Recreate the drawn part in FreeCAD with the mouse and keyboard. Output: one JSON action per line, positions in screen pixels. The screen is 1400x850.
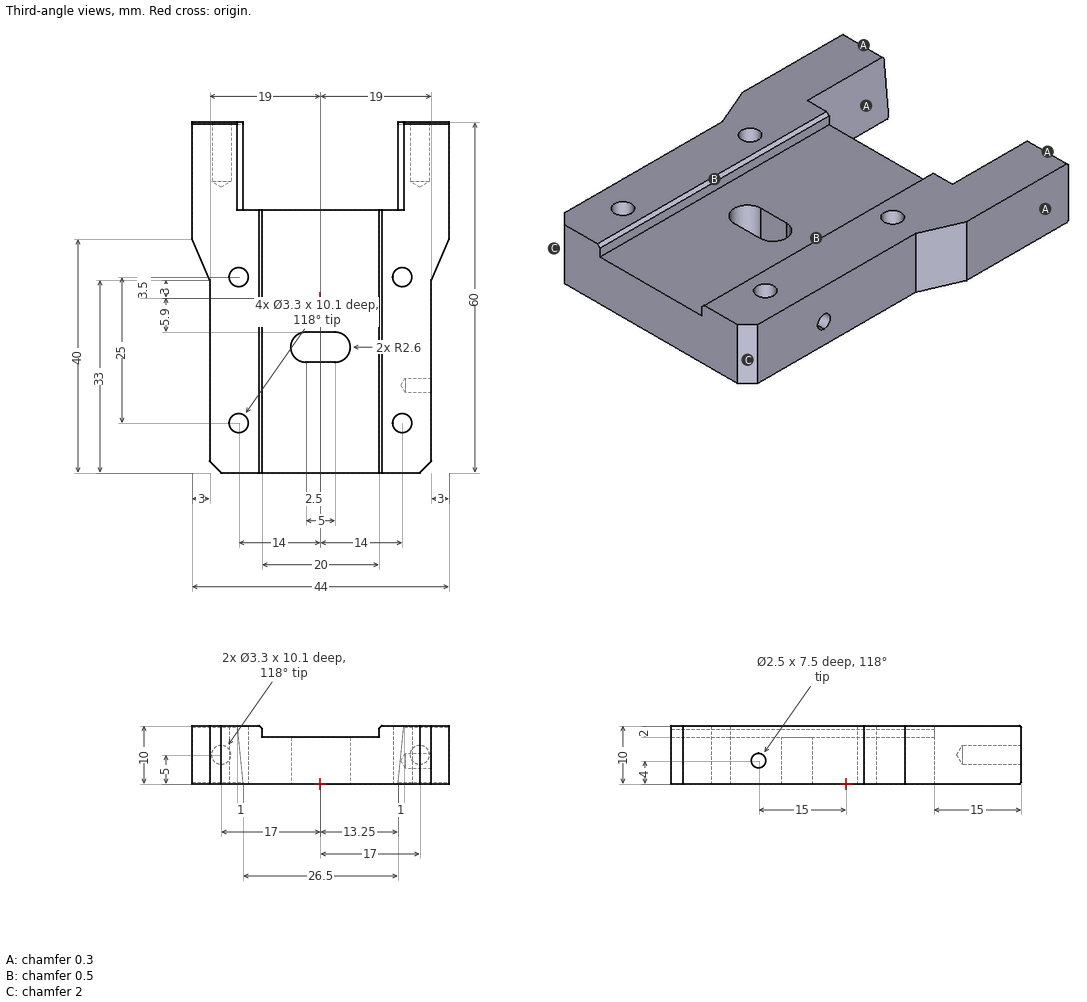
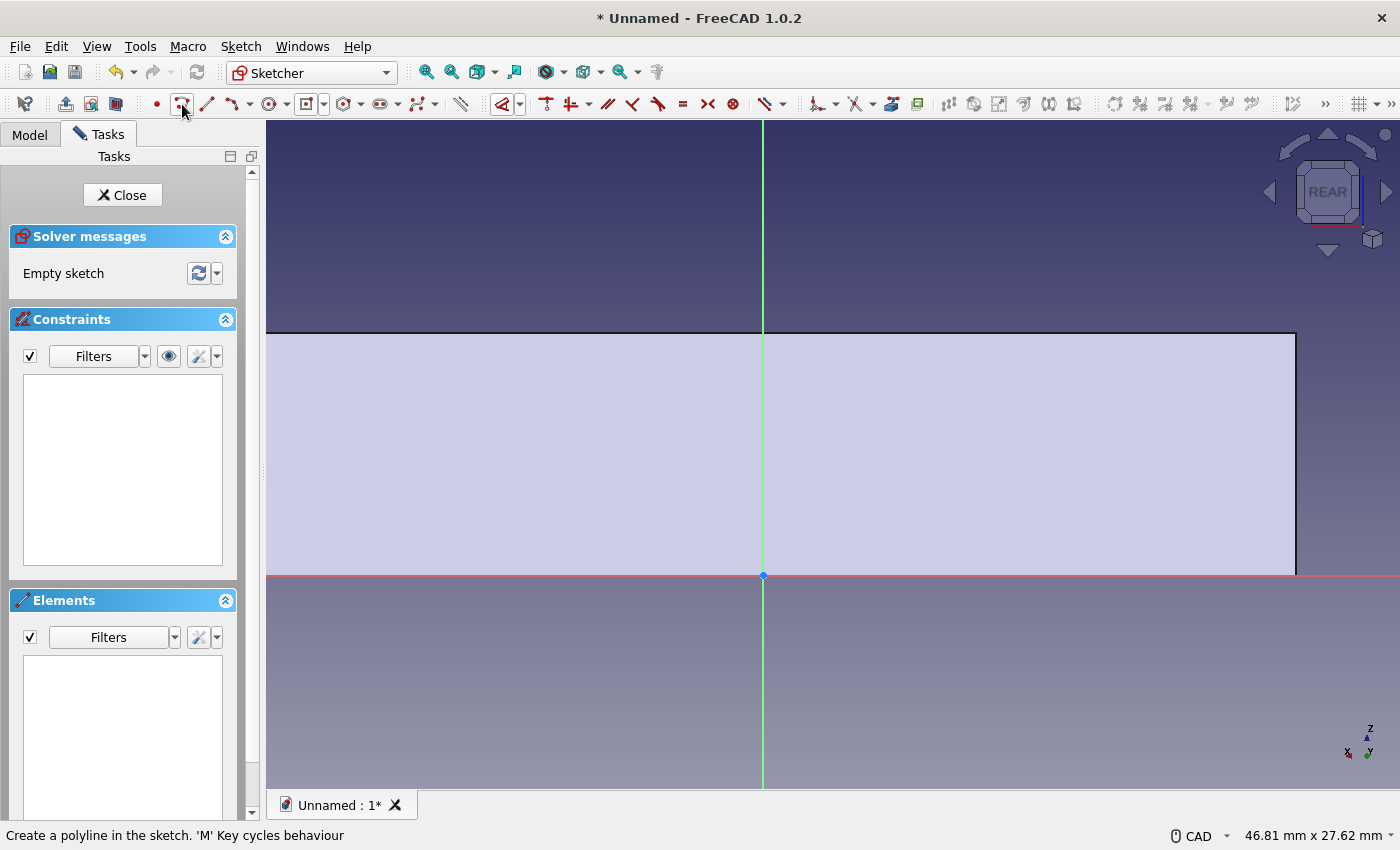
{"action": "left_click", "coordinate": [442, 576]}
{"action": "left_click", "coordinate": [1084, 567]}
{"action": "left_click", "coordinate": [1109, 333]}
{"action": "left_click", "coordinate": [418, 333]}
{"action": "left_click", "coordinate": [442, 576]}
{"action": "key", "text": "Escape"}
{"action": "key", "text": "Escape"}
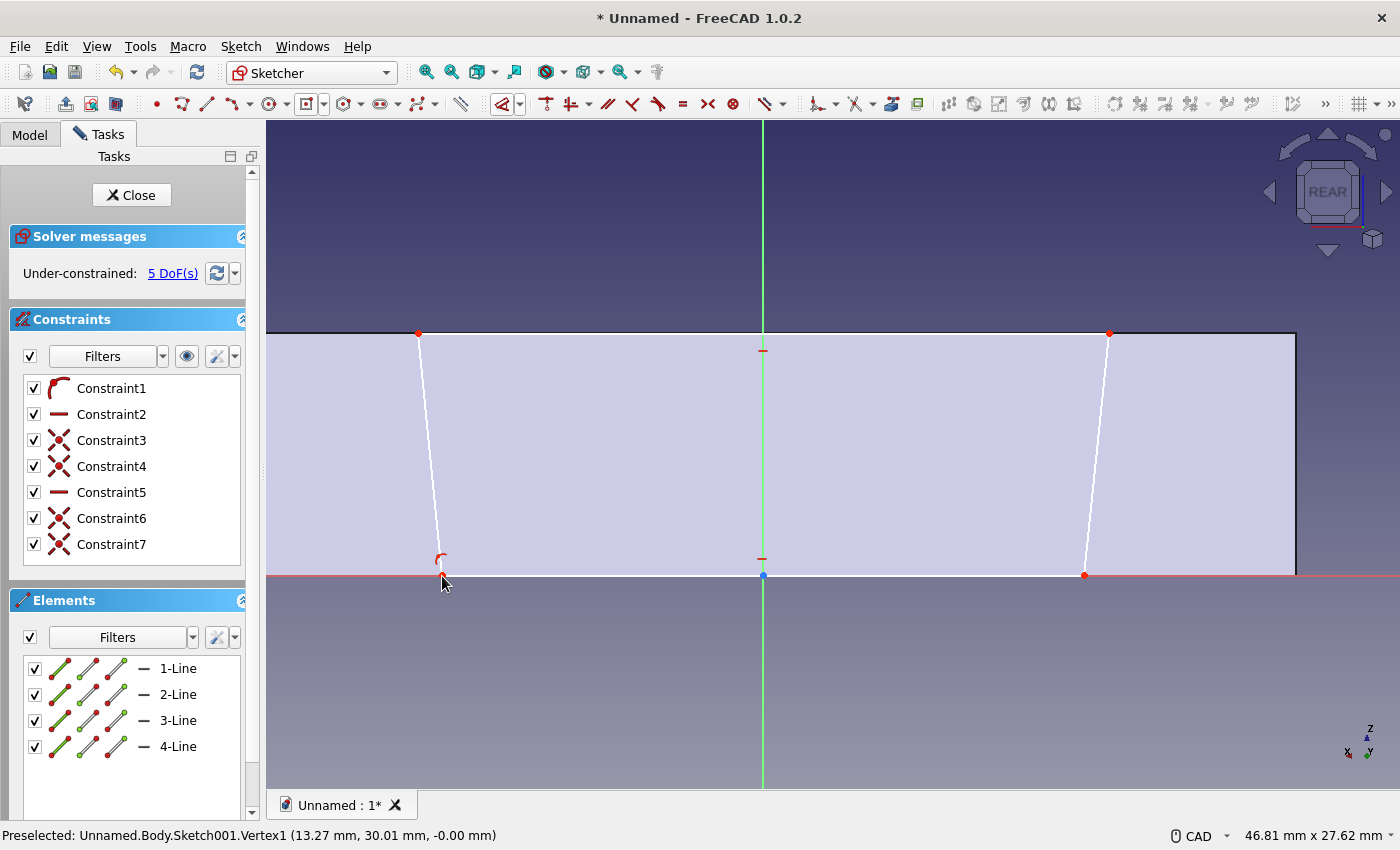
{"action": "scroll", "coordinate": [1091, 503], "scroll_direction": "up", "scroll_amount": 3}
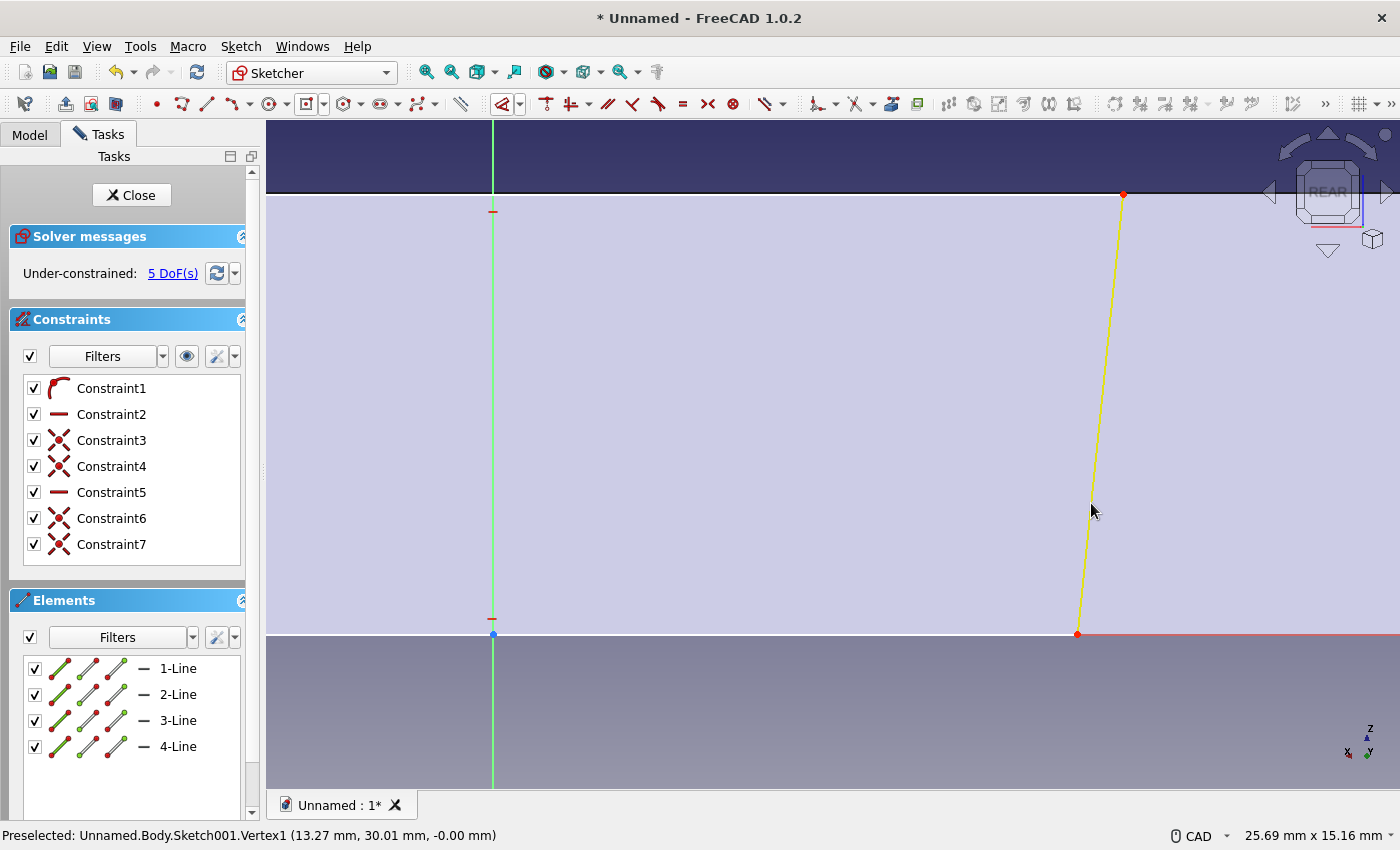
{"action": "left_click", "coordinate": [1091, 503]}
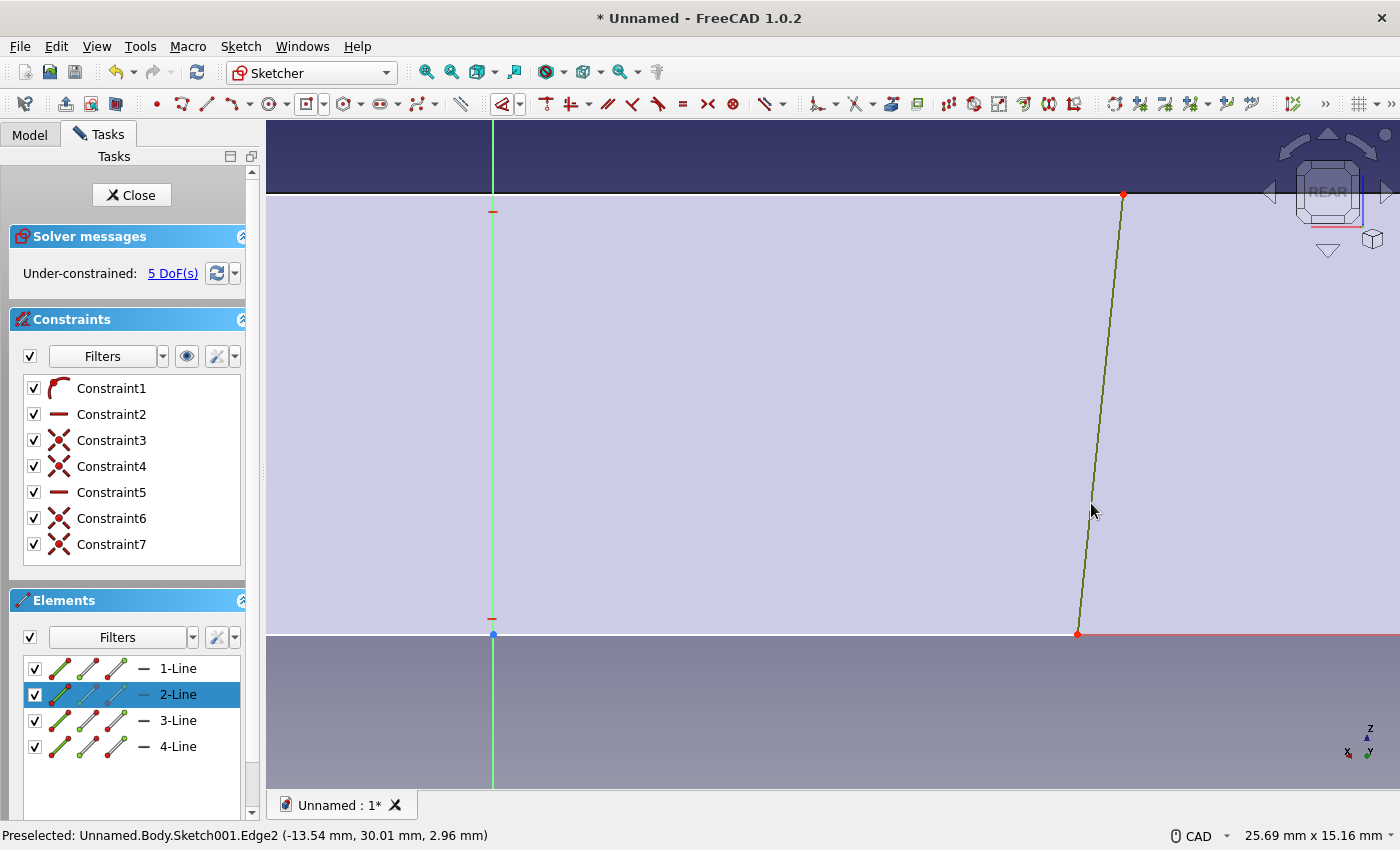
{"action": "key", "text": "l"}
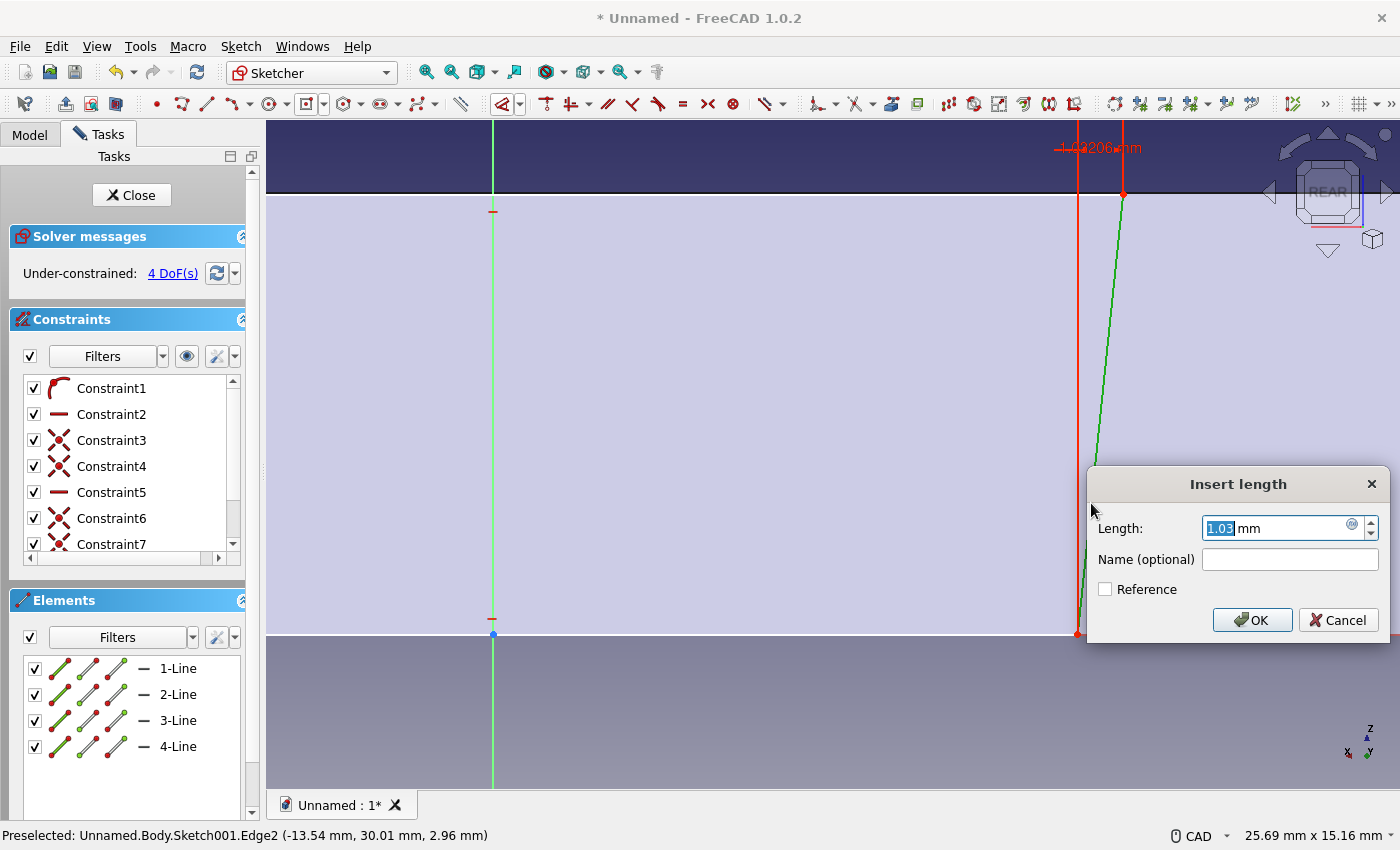
{"action": "type", "text": "1"}
{"action": "key", "text": "Return"}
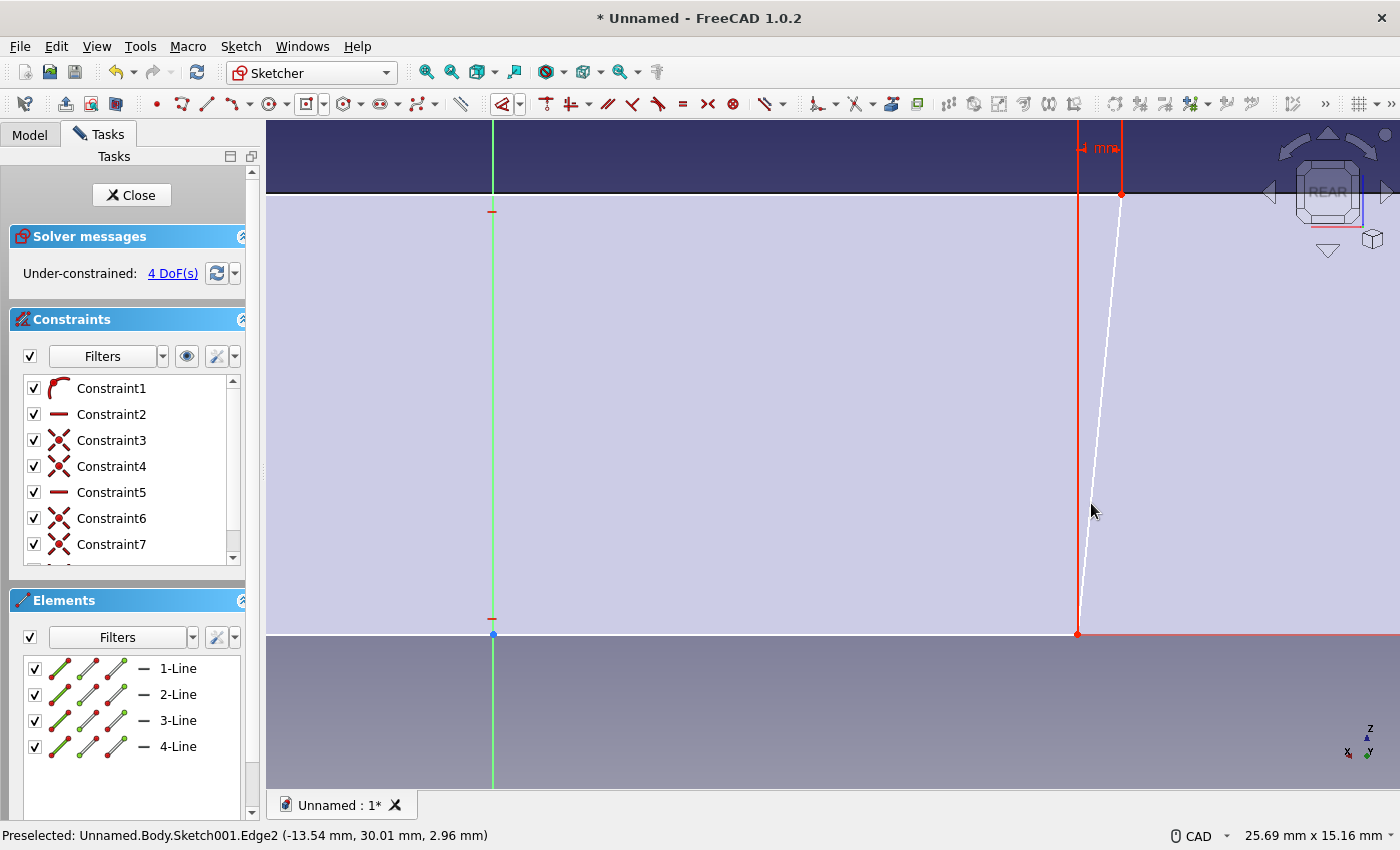
{"action": "scroll", "coordinate": [1094, 504], "scroll_direction": "down", "scroll_amount": 3}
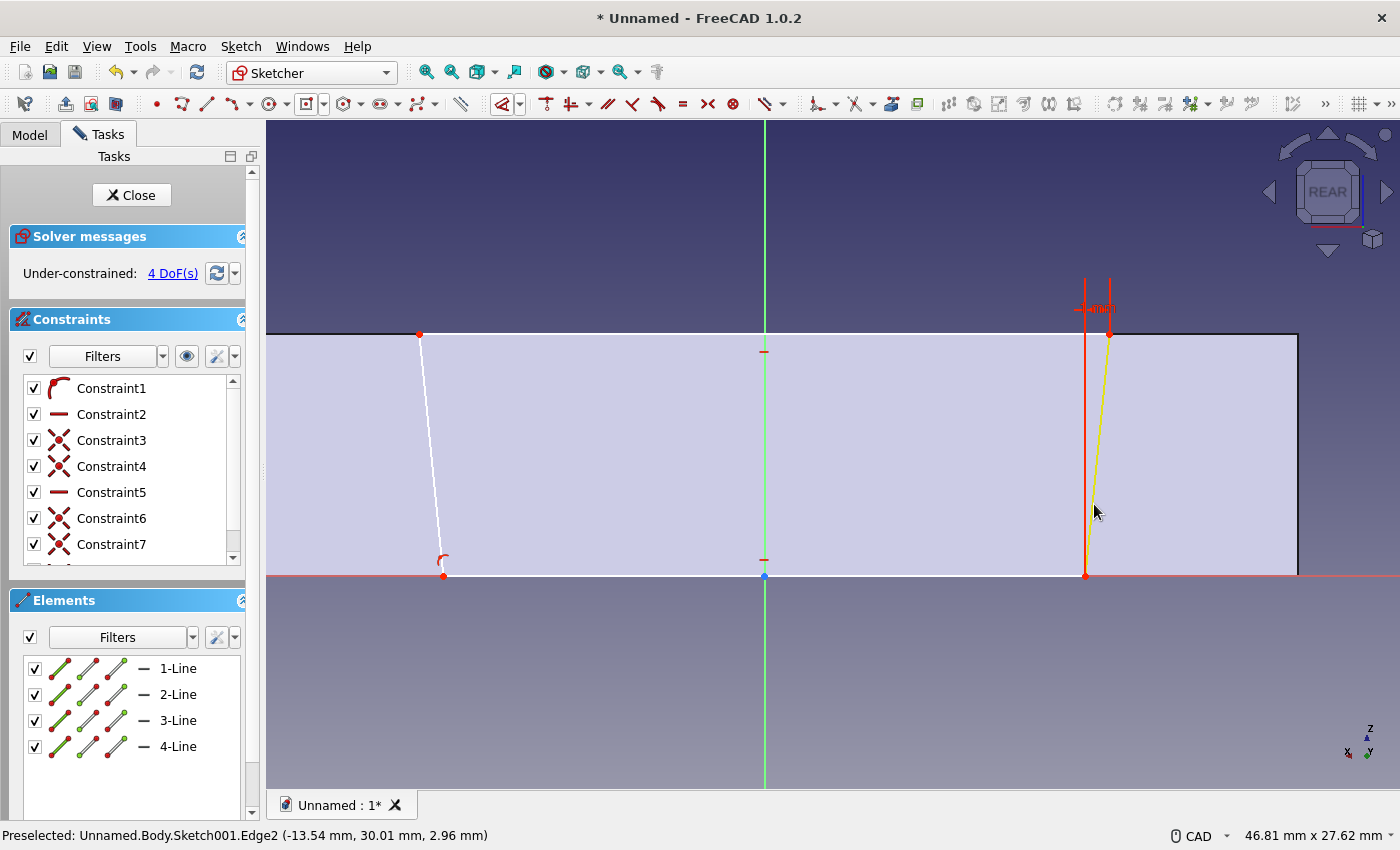
{"action": "scroll", "coordinate": [427, 407], "scroll_direction": "up", "scroll_amount": 3}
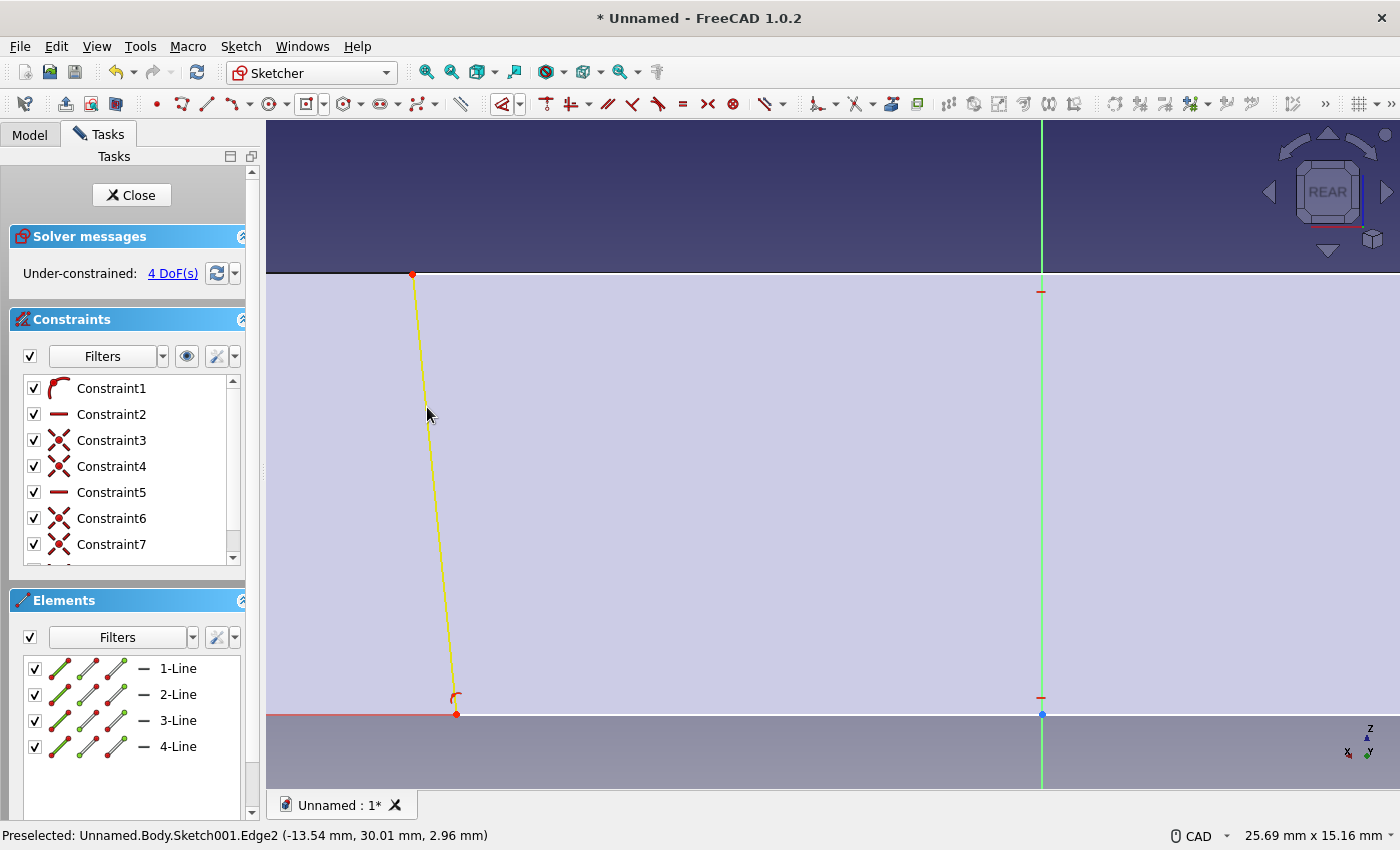
{"action": "left_click", "coordinate": [426, 407]}